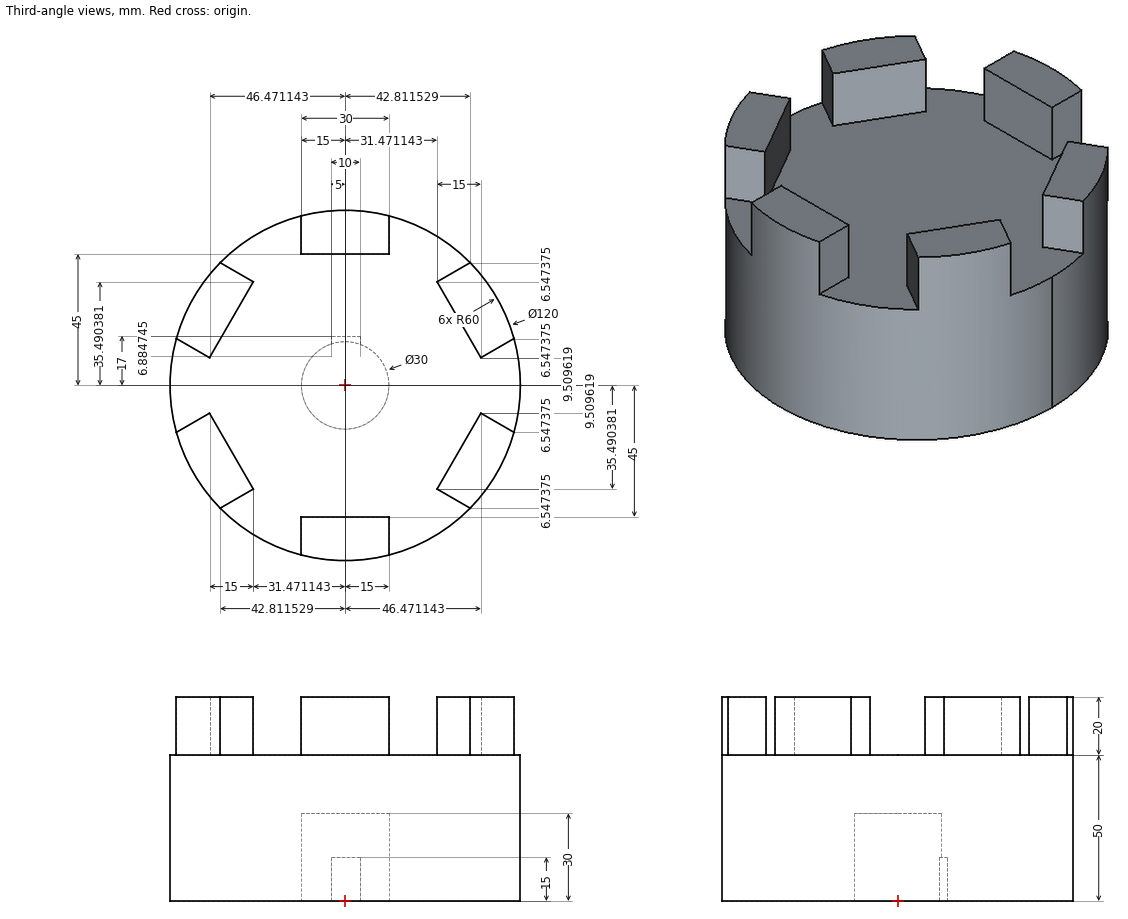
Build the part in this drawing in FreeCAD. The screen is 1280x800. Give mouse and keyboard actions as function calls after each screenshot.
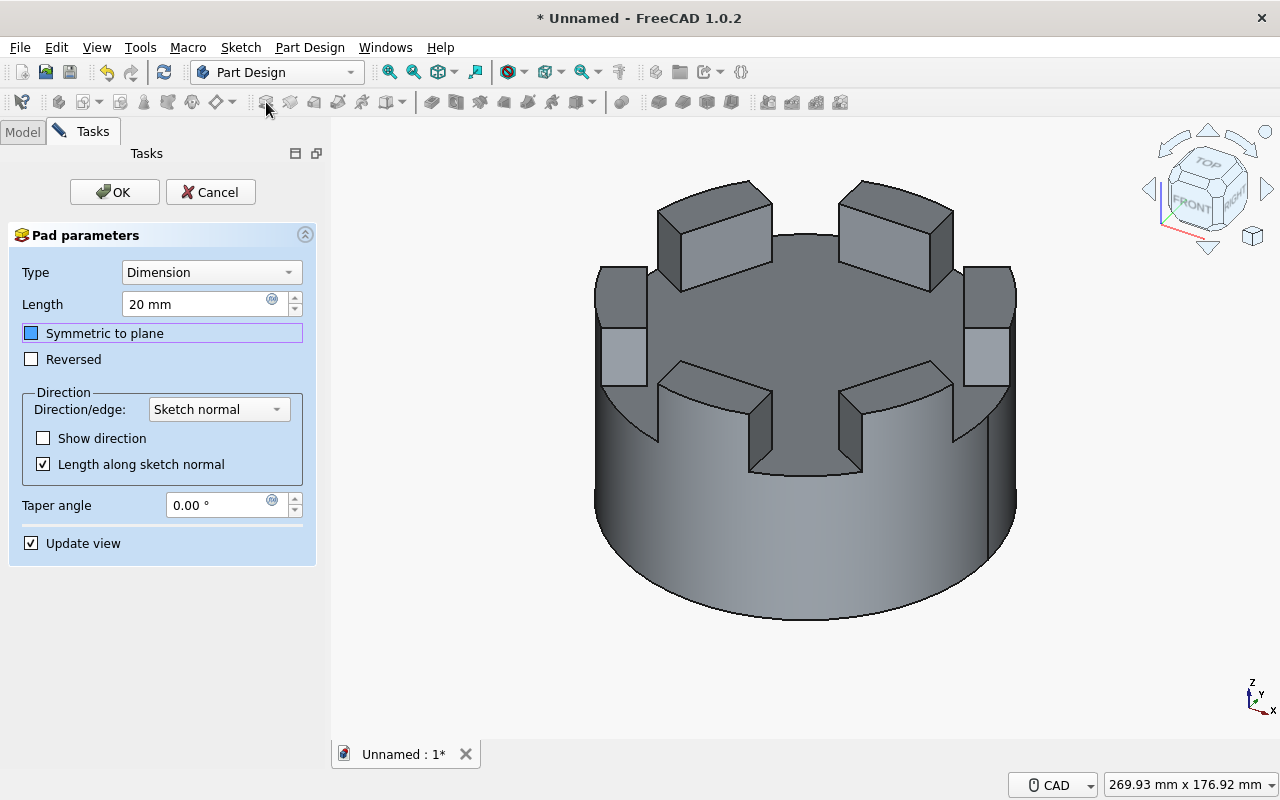
click(115, 192)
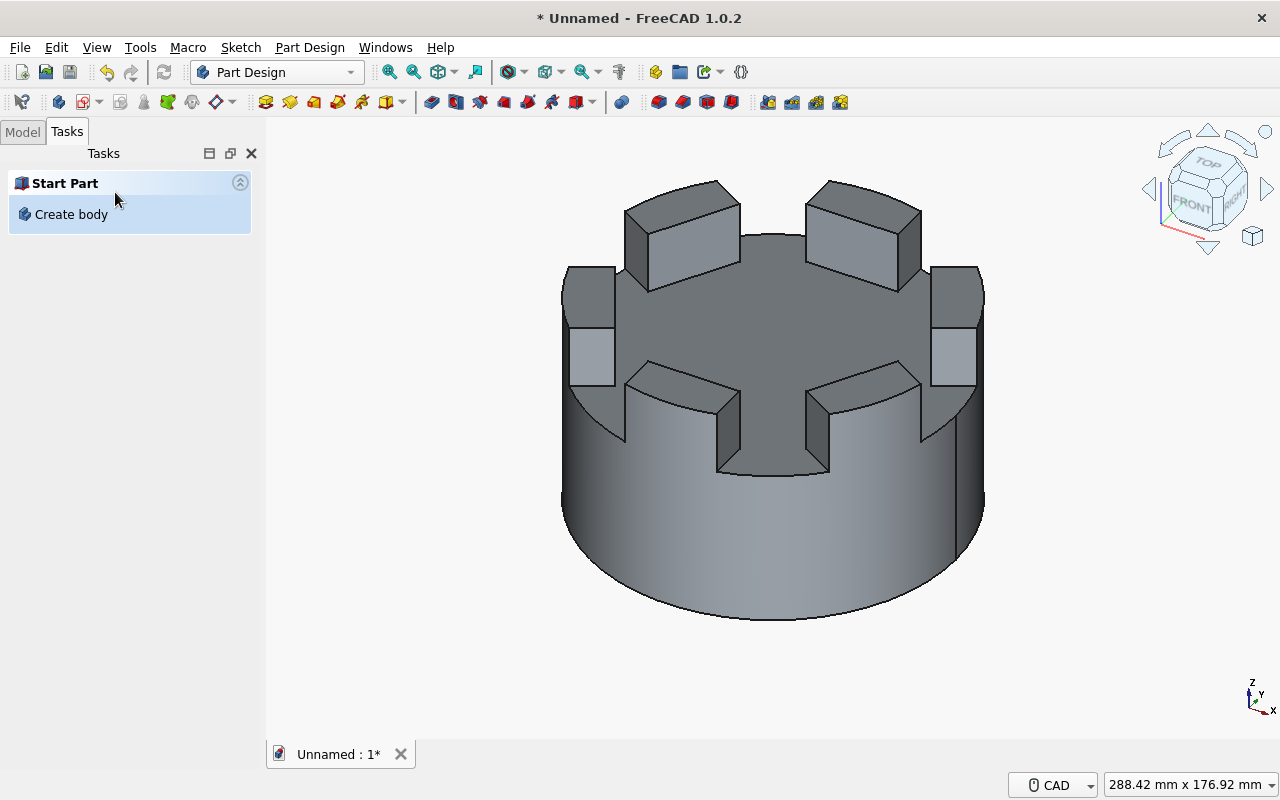
click(84, 102)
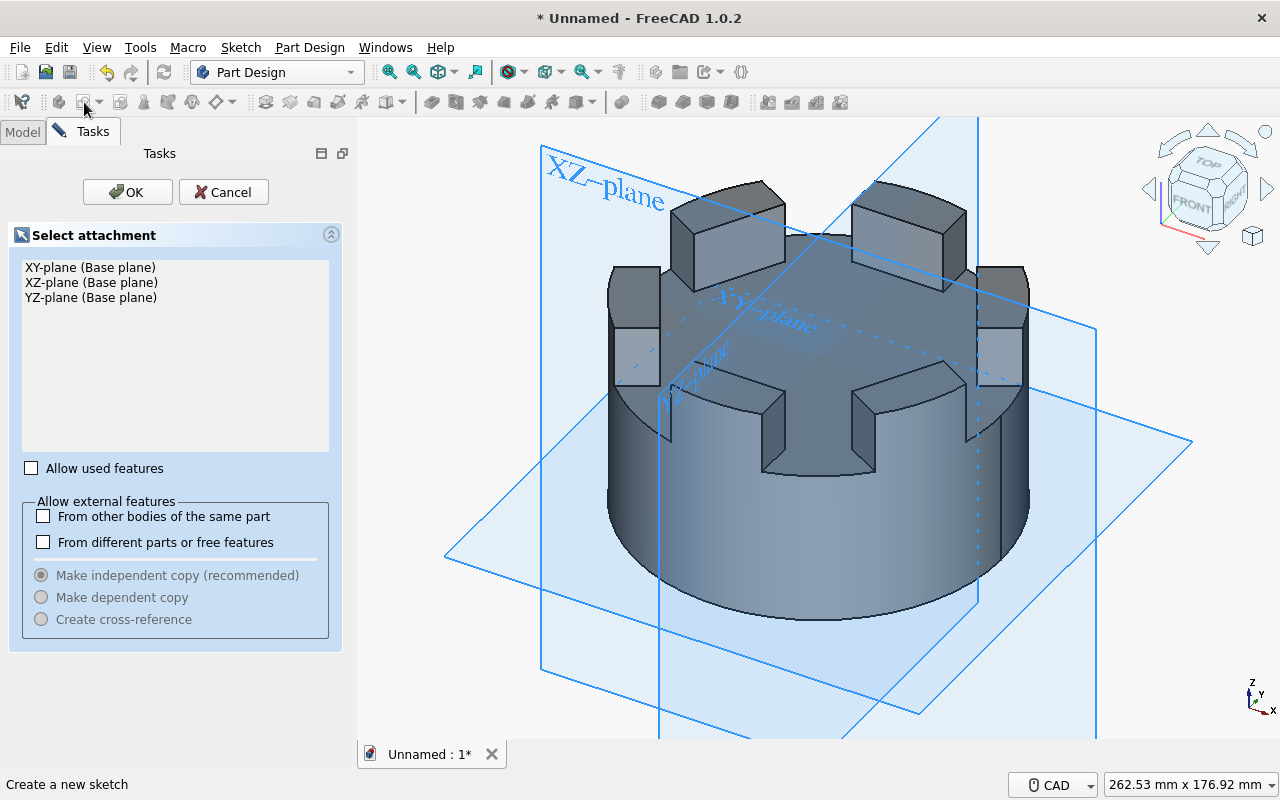
click(82, 268)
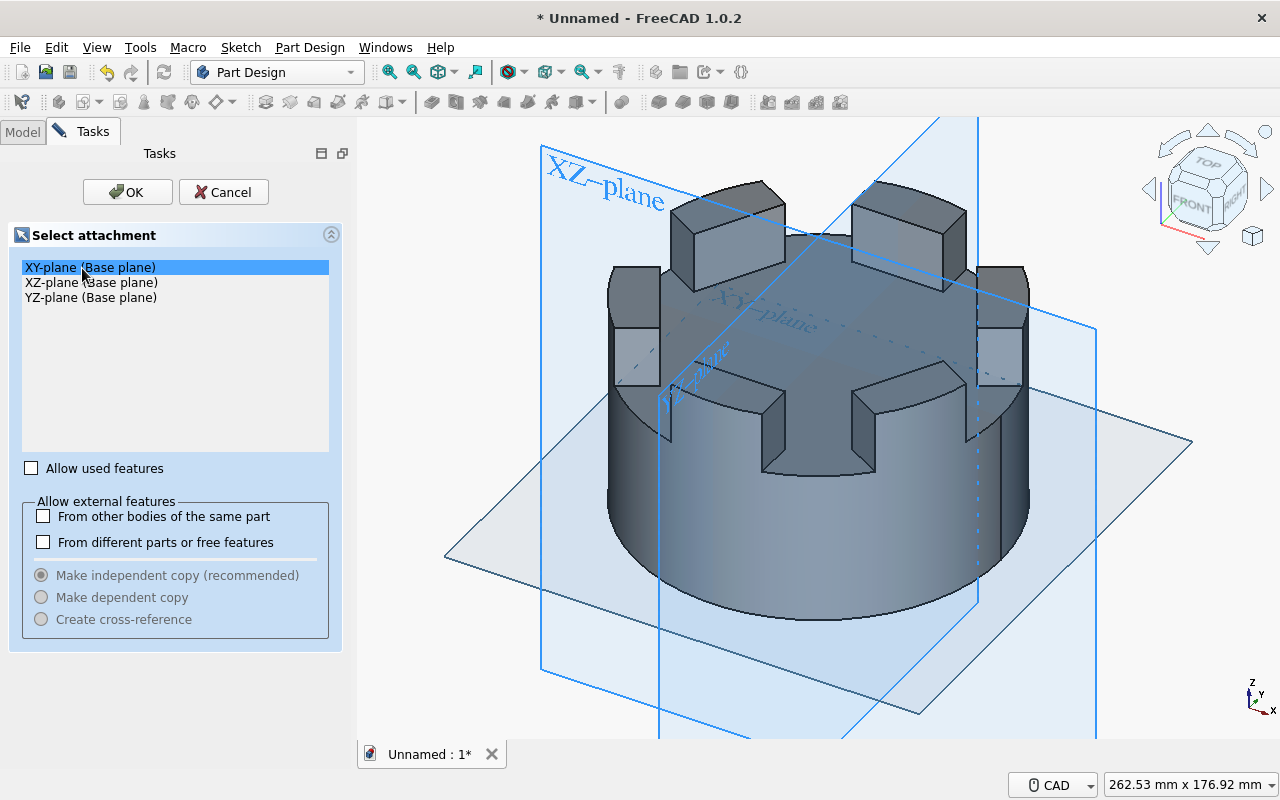
click(128, 192)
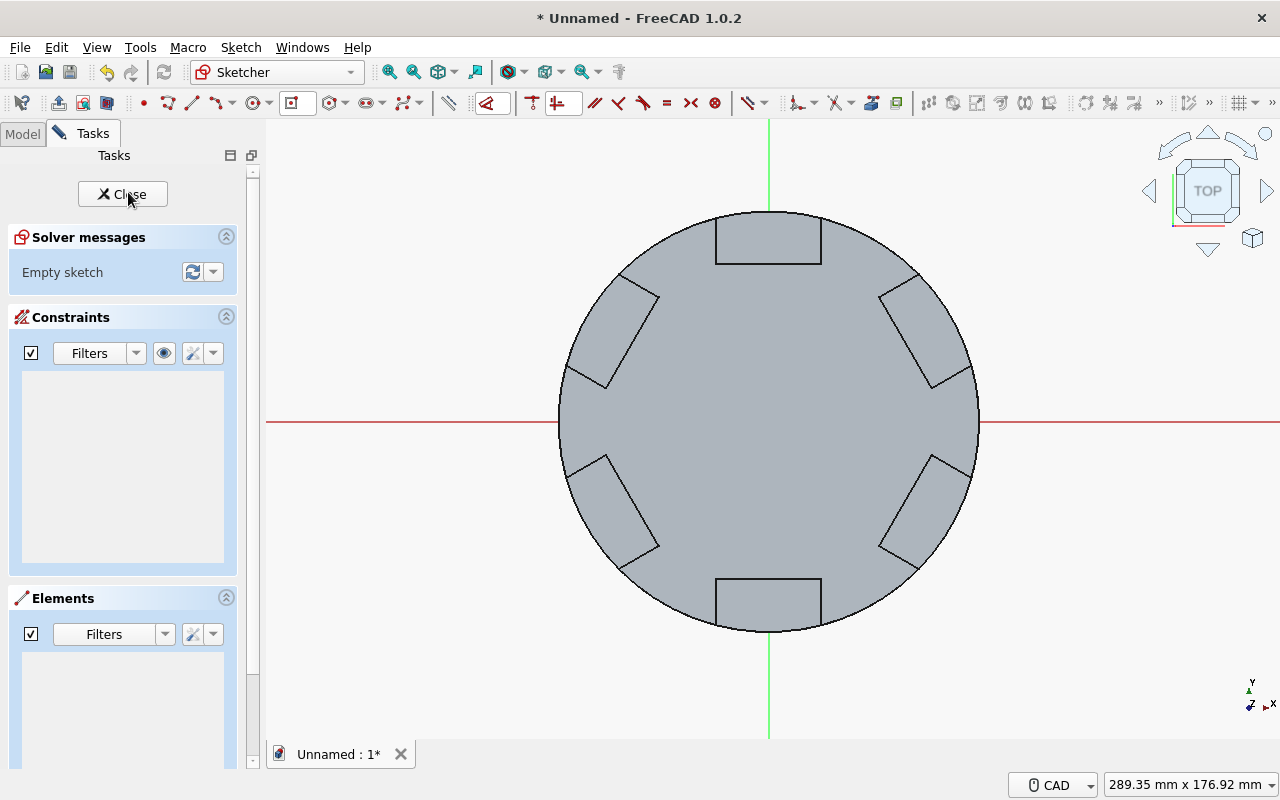
key(q)
key(s)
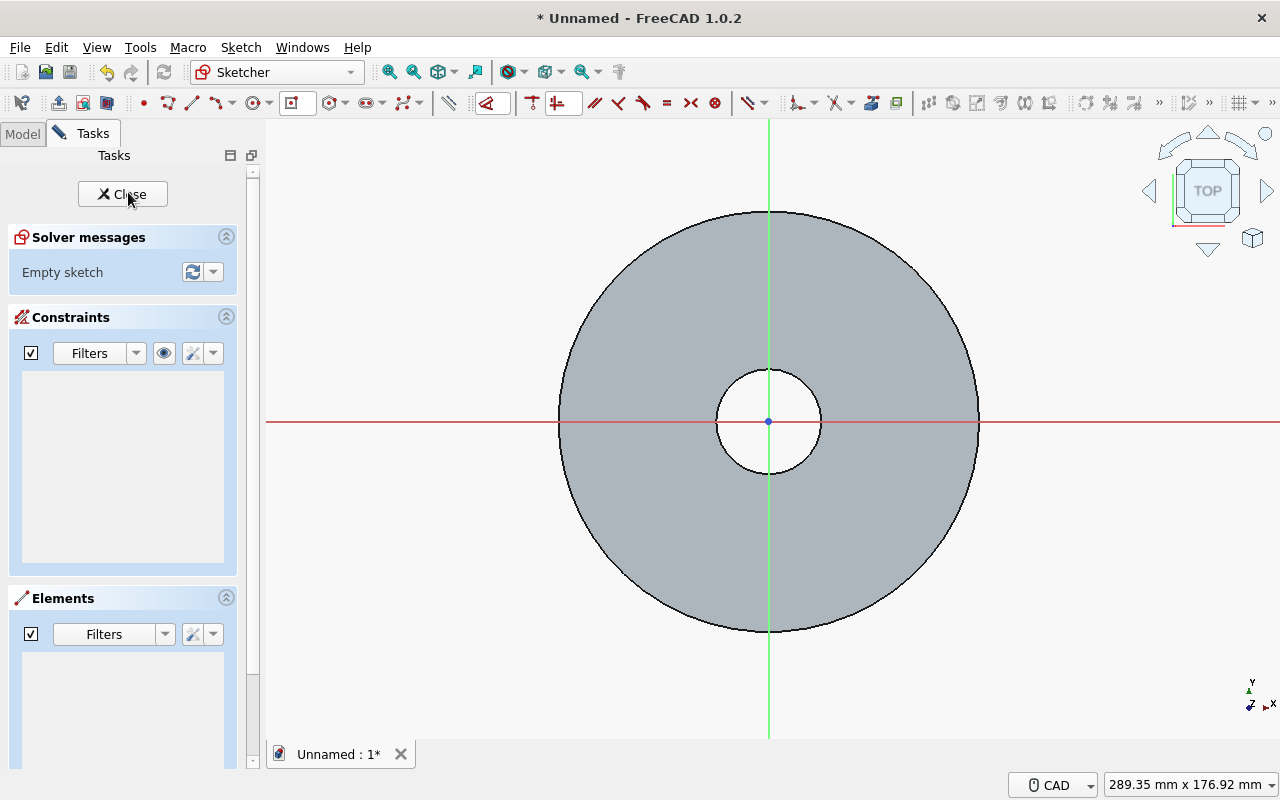
scroll(782, 385, up, 9)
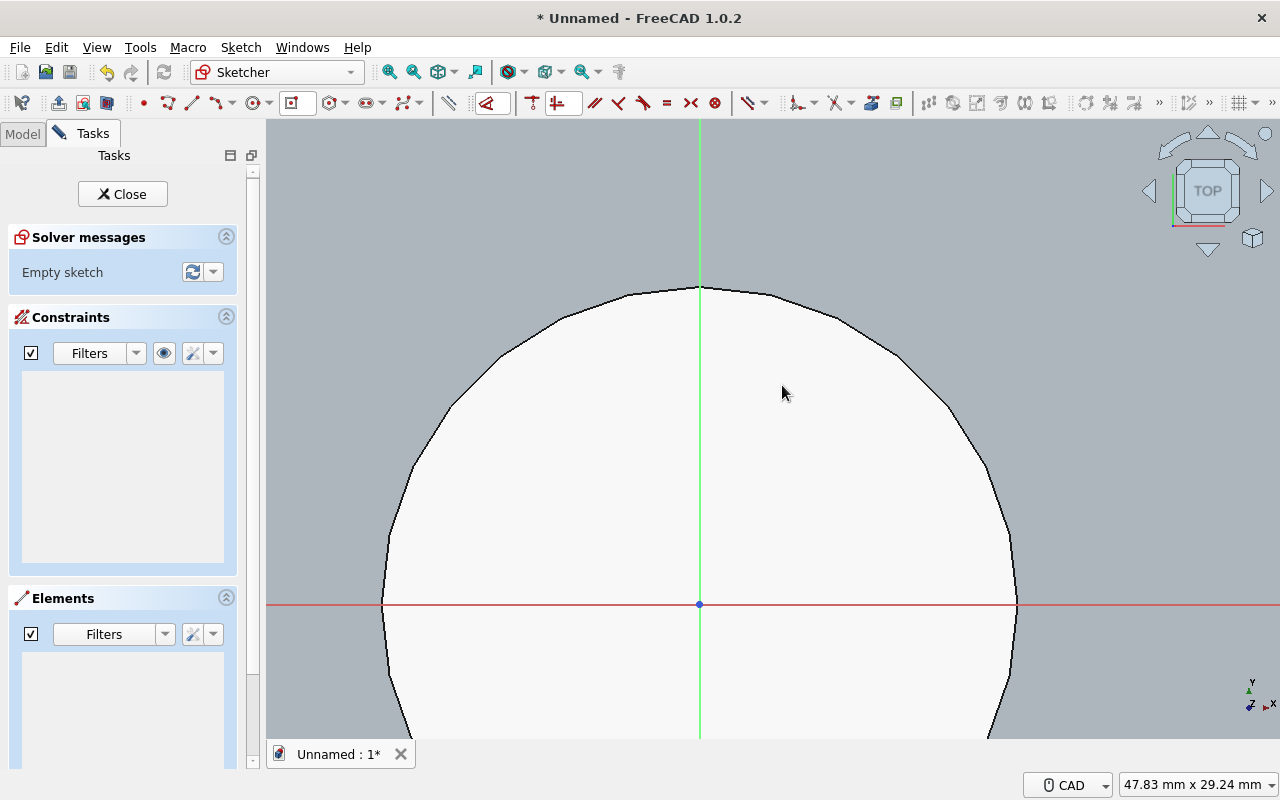
key(g)
key(r)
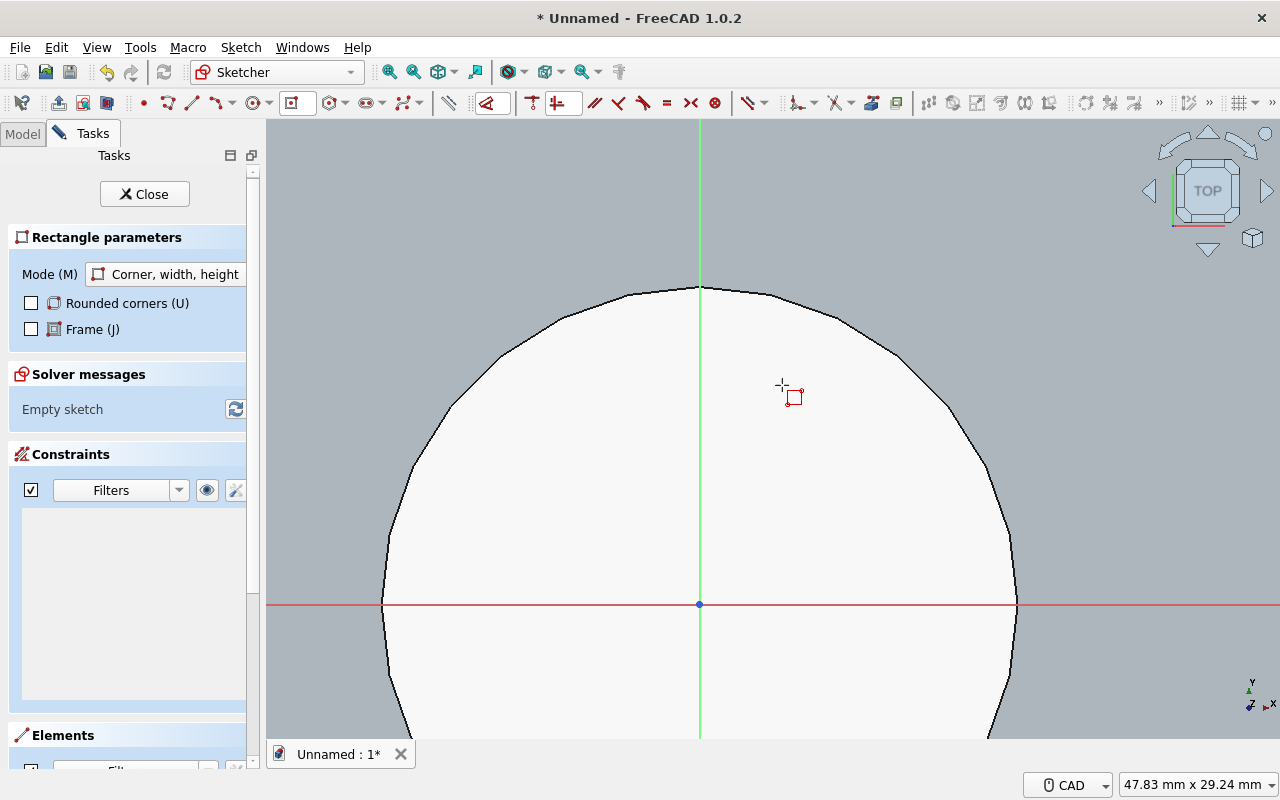
click(594, 245)
click(806, 391)
key(Escape)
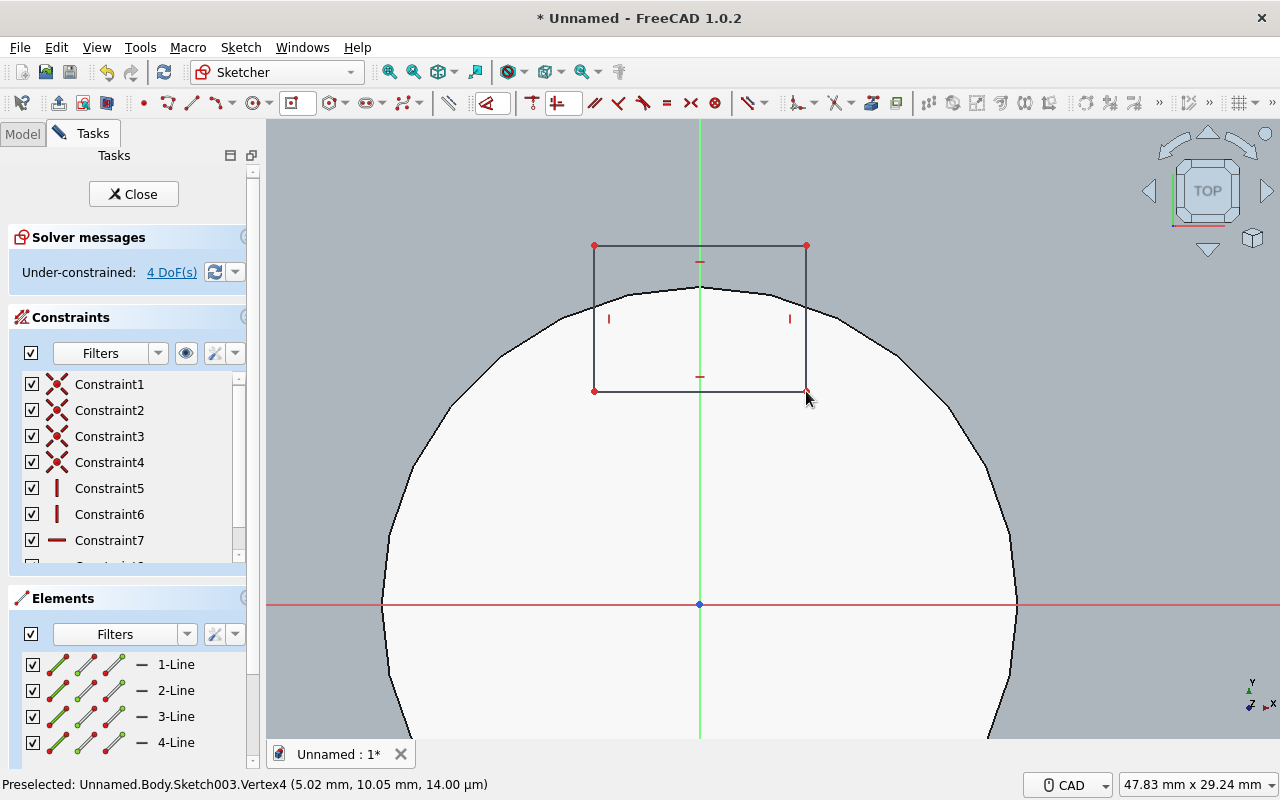
click(658, 392)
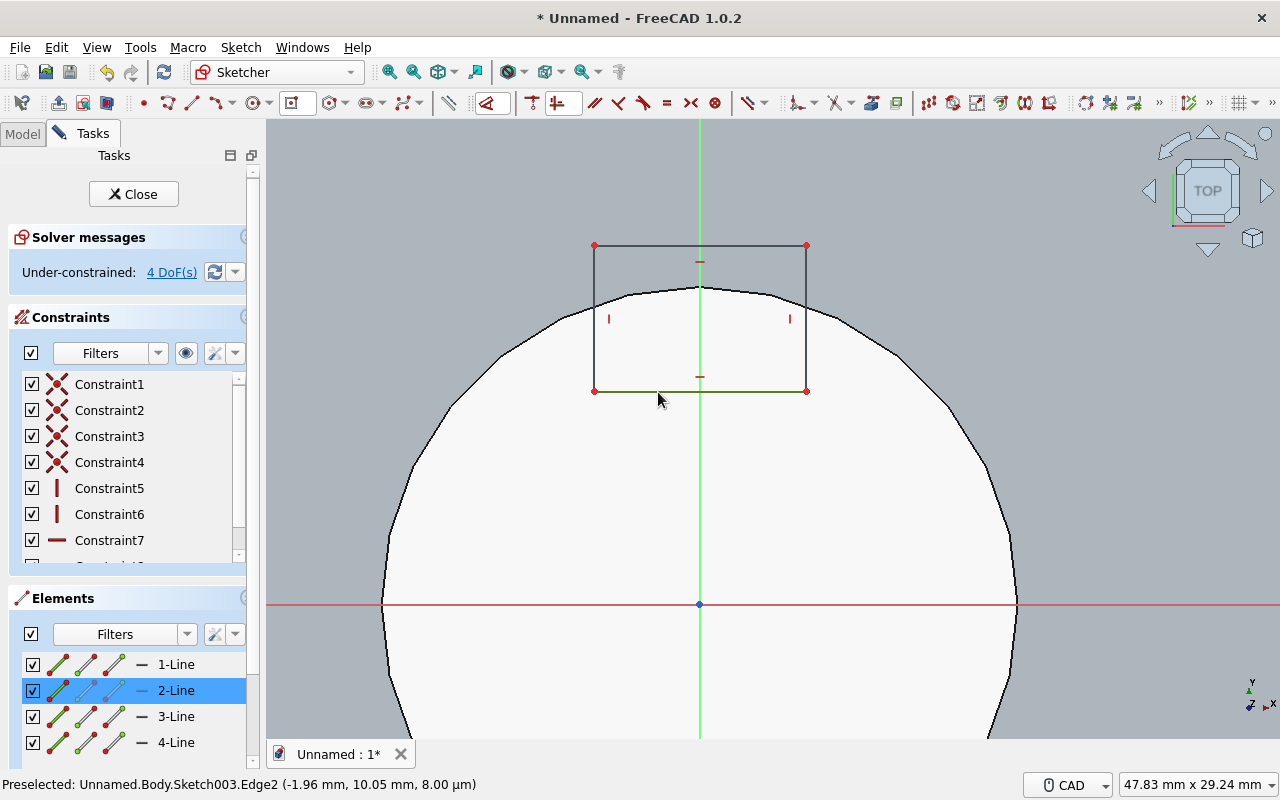
key(l)